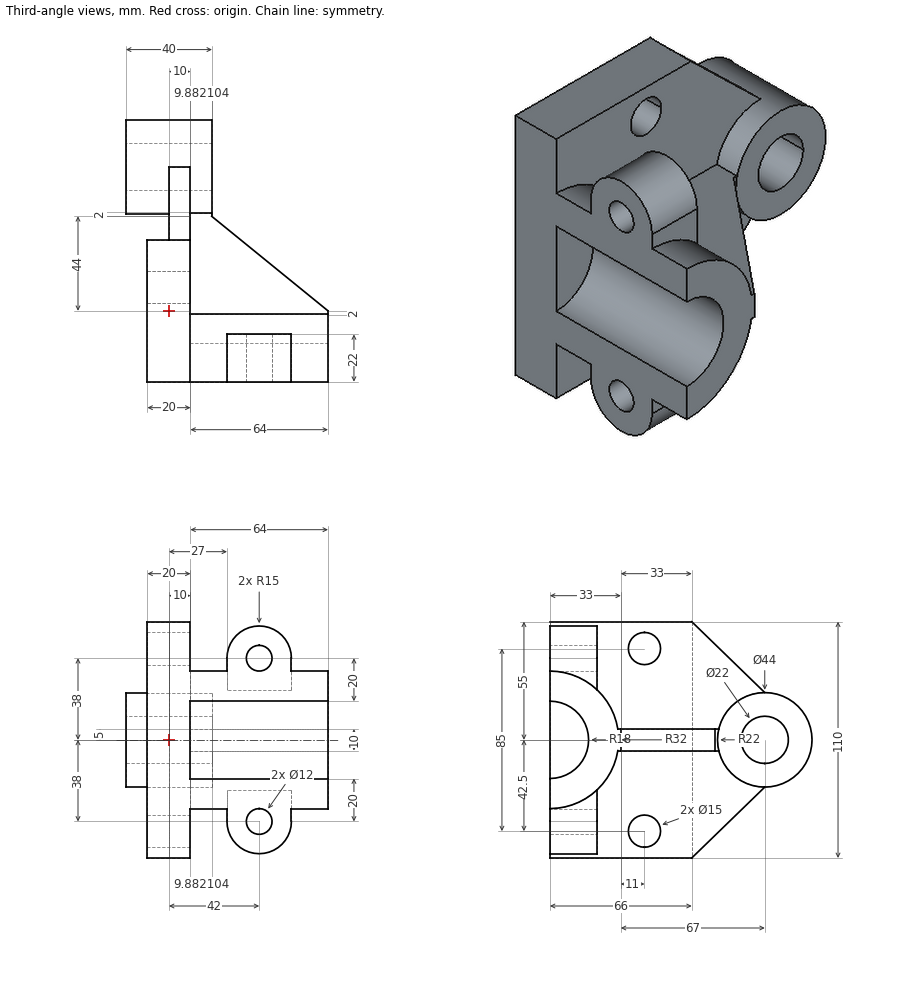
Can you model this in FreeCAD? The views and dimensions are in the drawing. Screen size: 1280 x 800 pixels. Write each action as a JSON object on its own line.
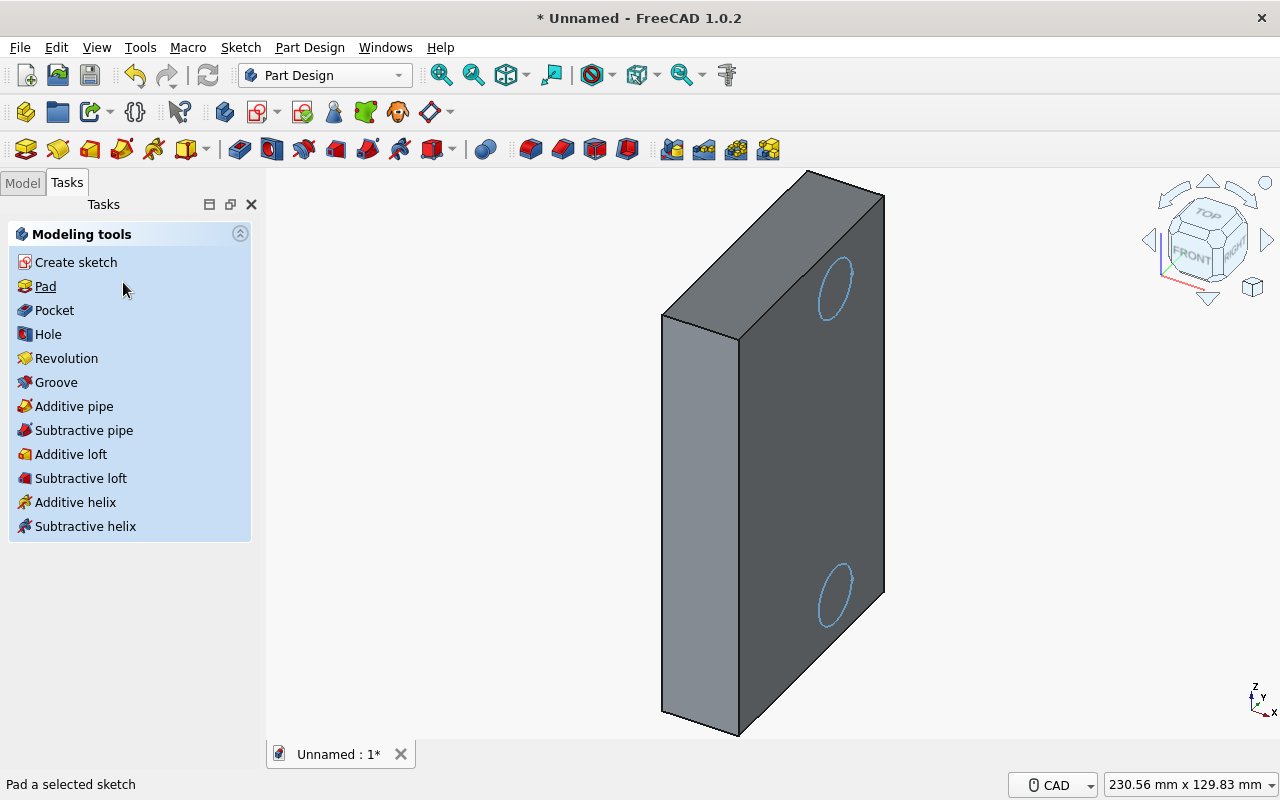
{"action": "left_click", "coordinate": [240, 150]}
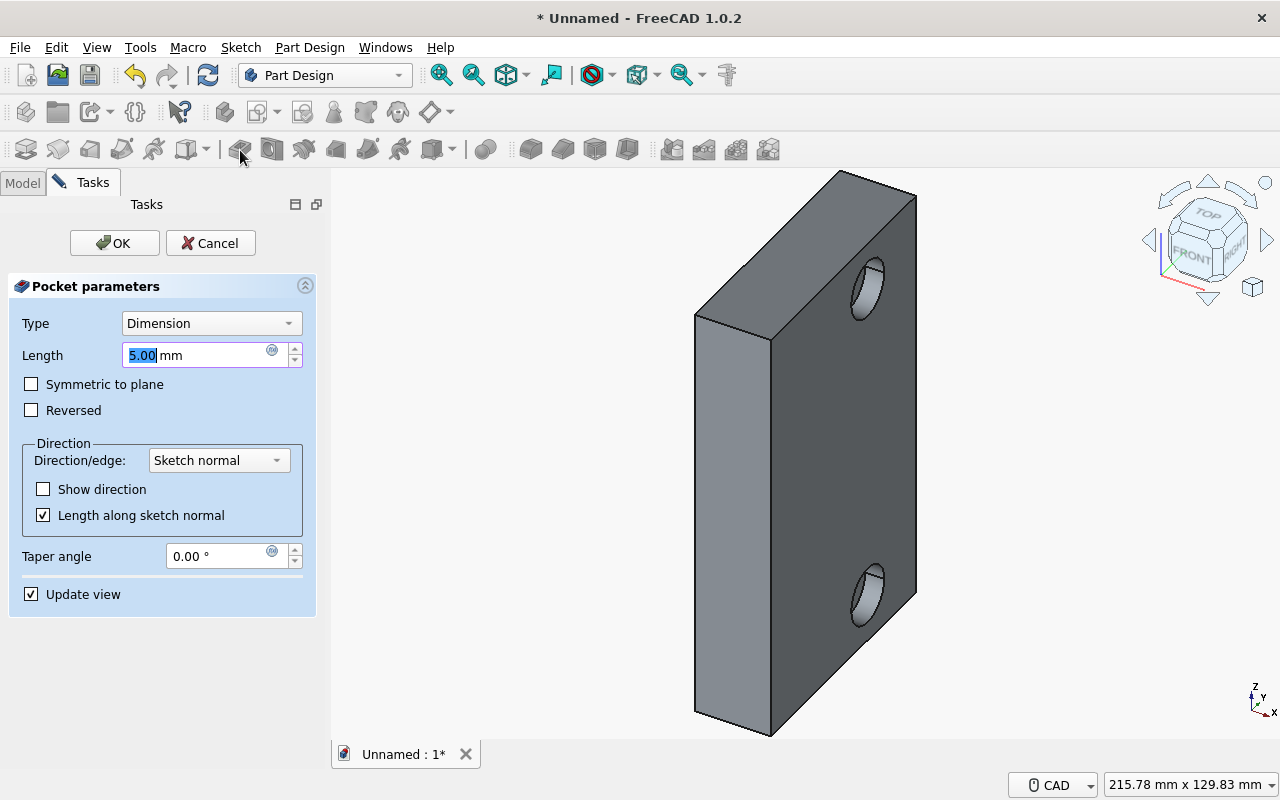
{"action": "type", "text": "20"}
{"action": "key", "text": "Tab"}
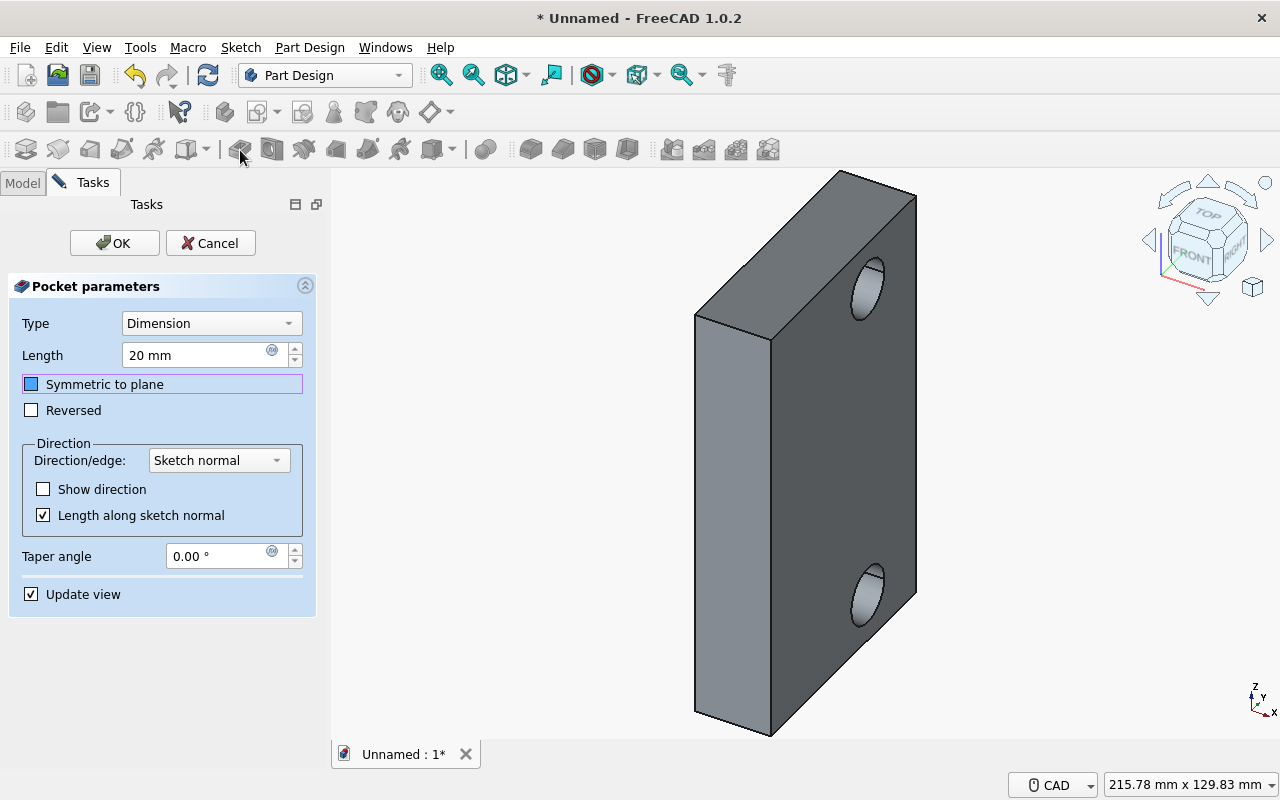
{"action": "left_click", "coordinate": [115, 243]}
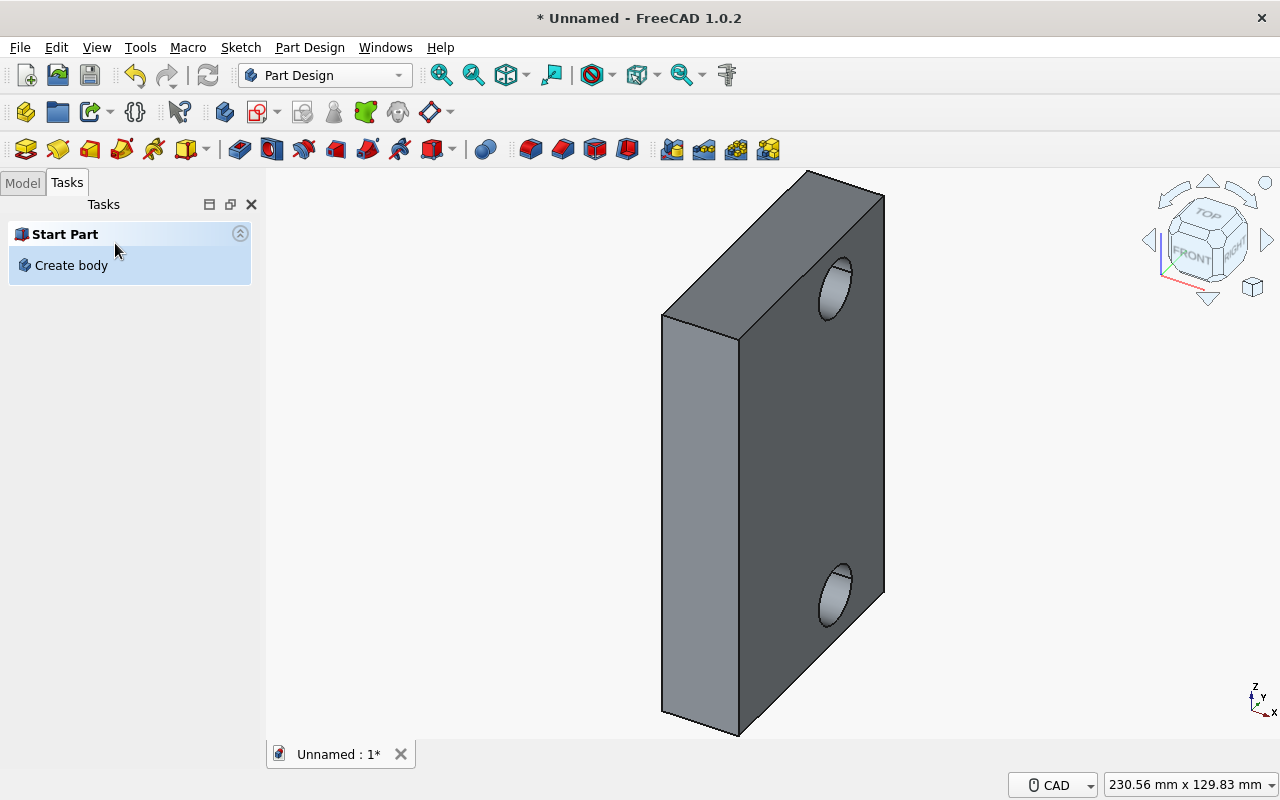
{"action": "left_click", "coordinate": [811, 465]}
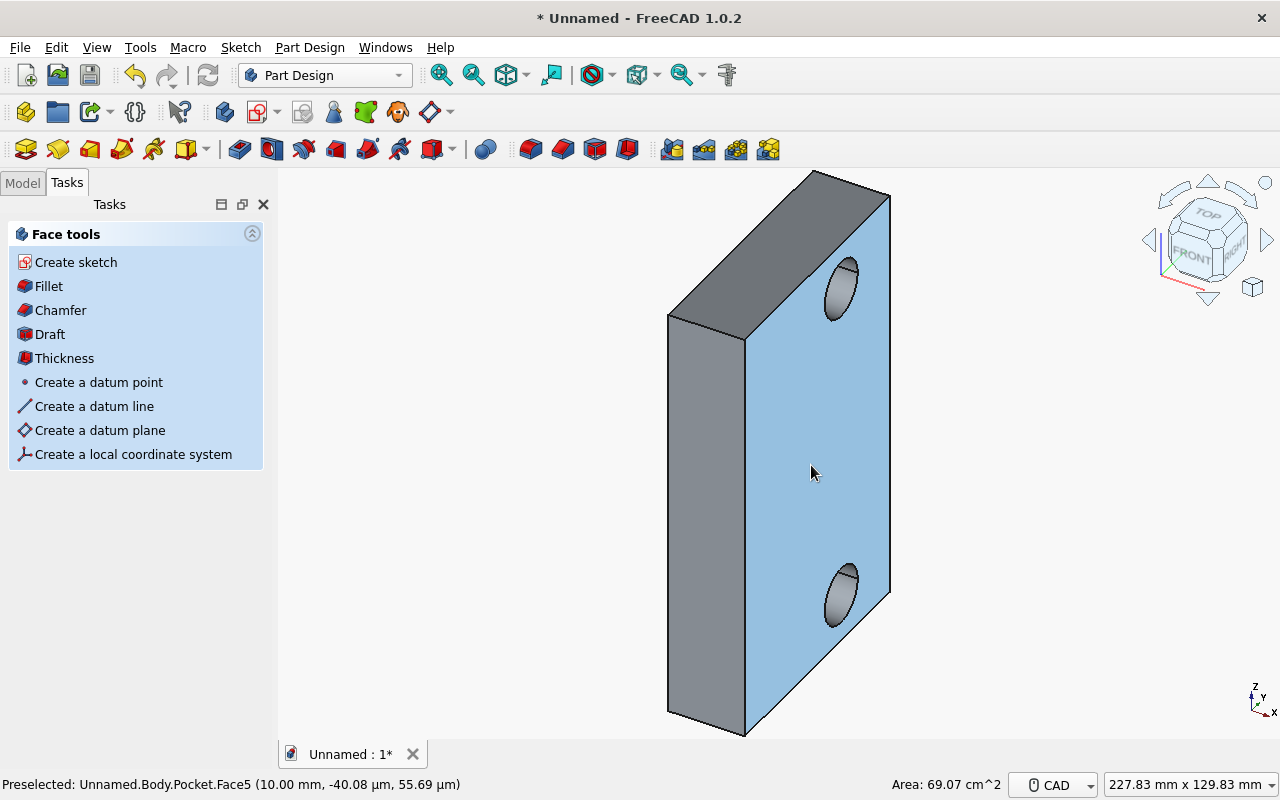
{"action": "left_click", "coordinate": [258, 112]}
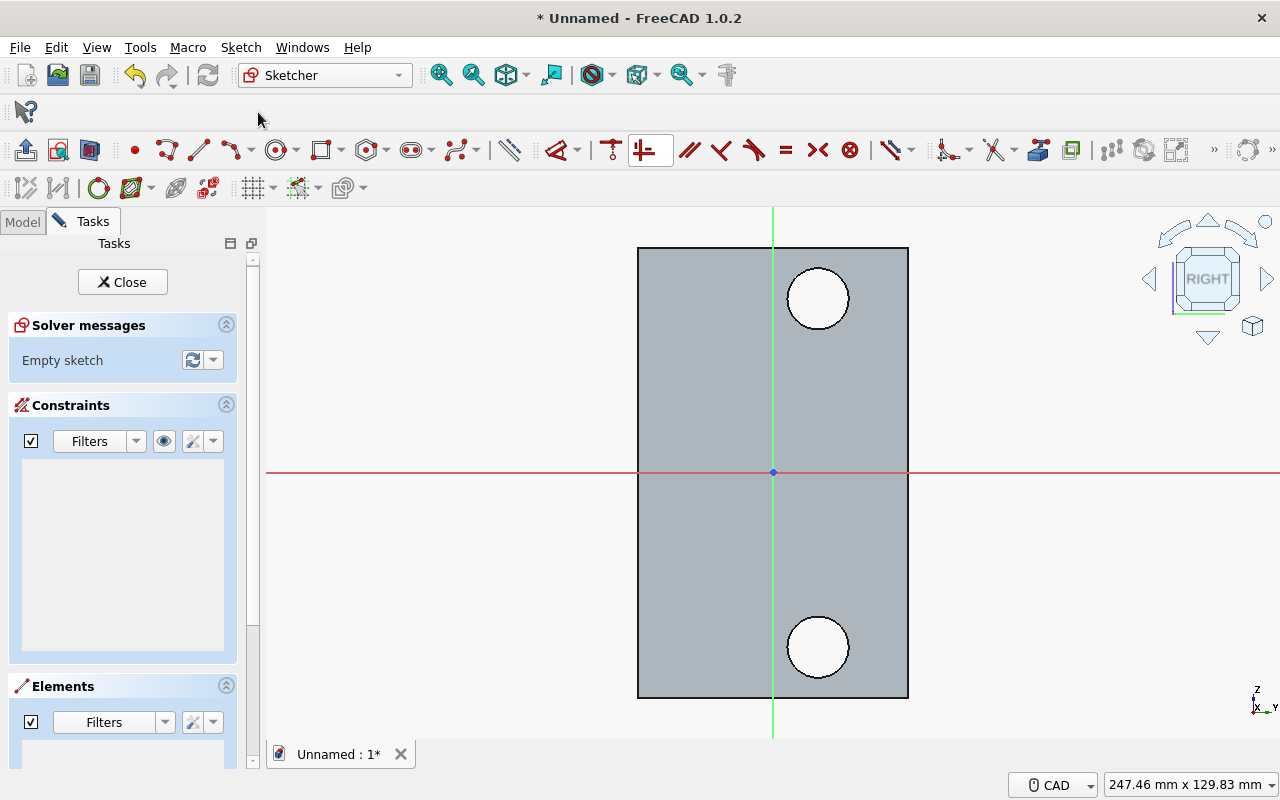
{"action": "key", "text": "g l"}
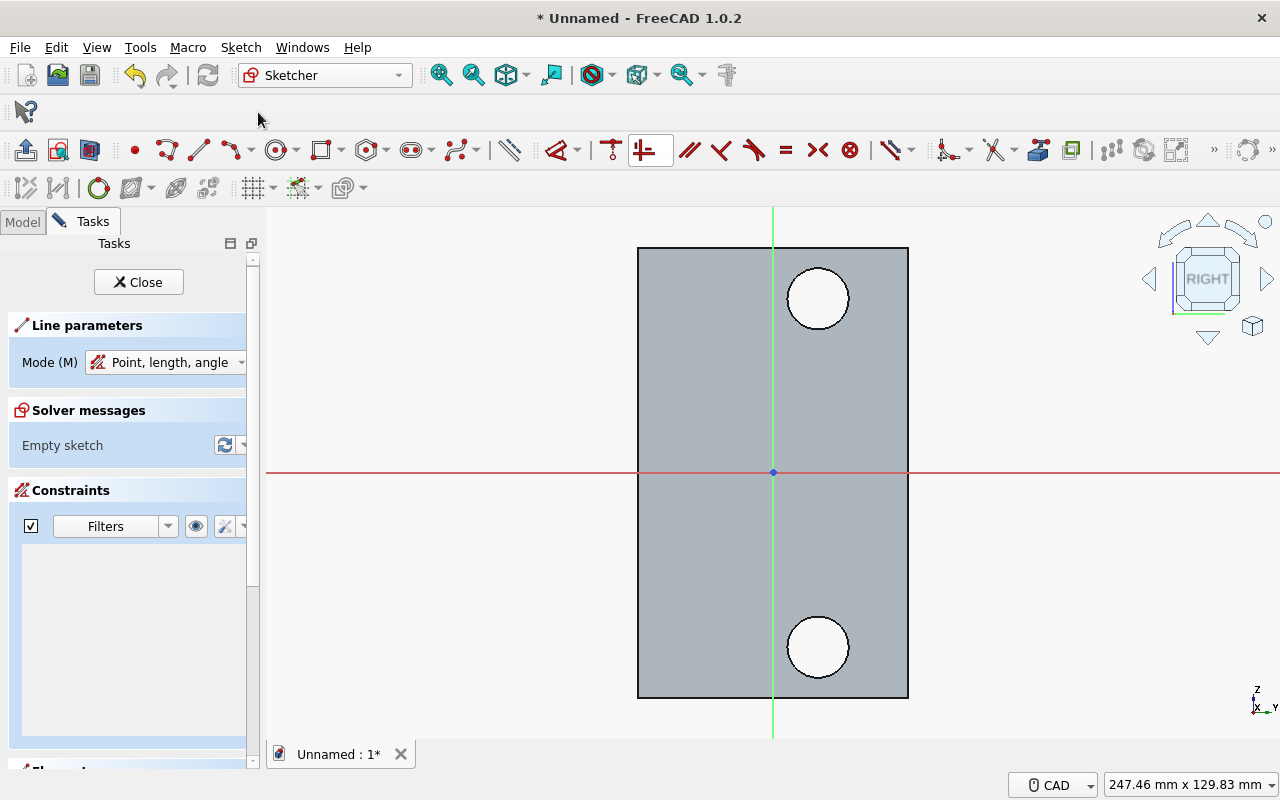
{"action": "left_click", "coordinate": [638, 342]}
{"action": "left_click", "coordinate": [638, 399]}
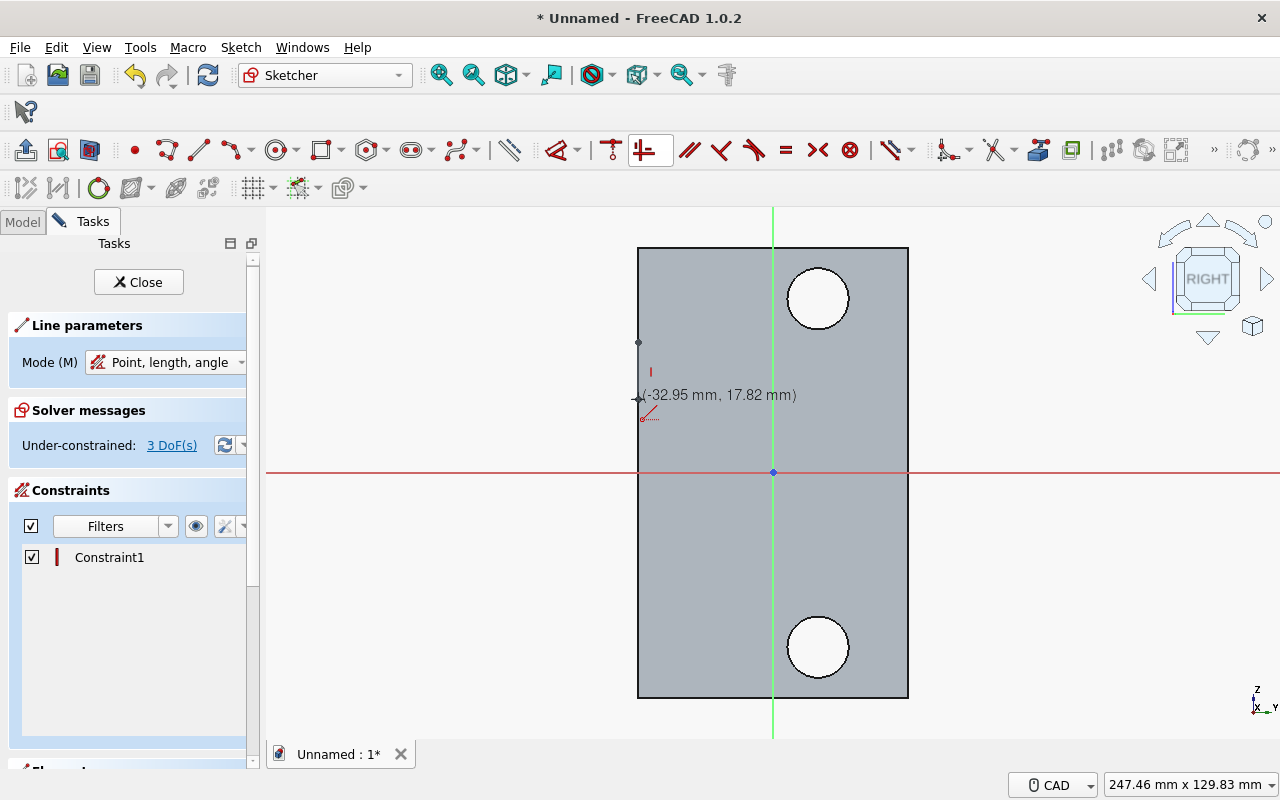
{"action": "left_click", "coordinate": [638, 547]}
{"action": "left_click", "coordinate": [638, 604]}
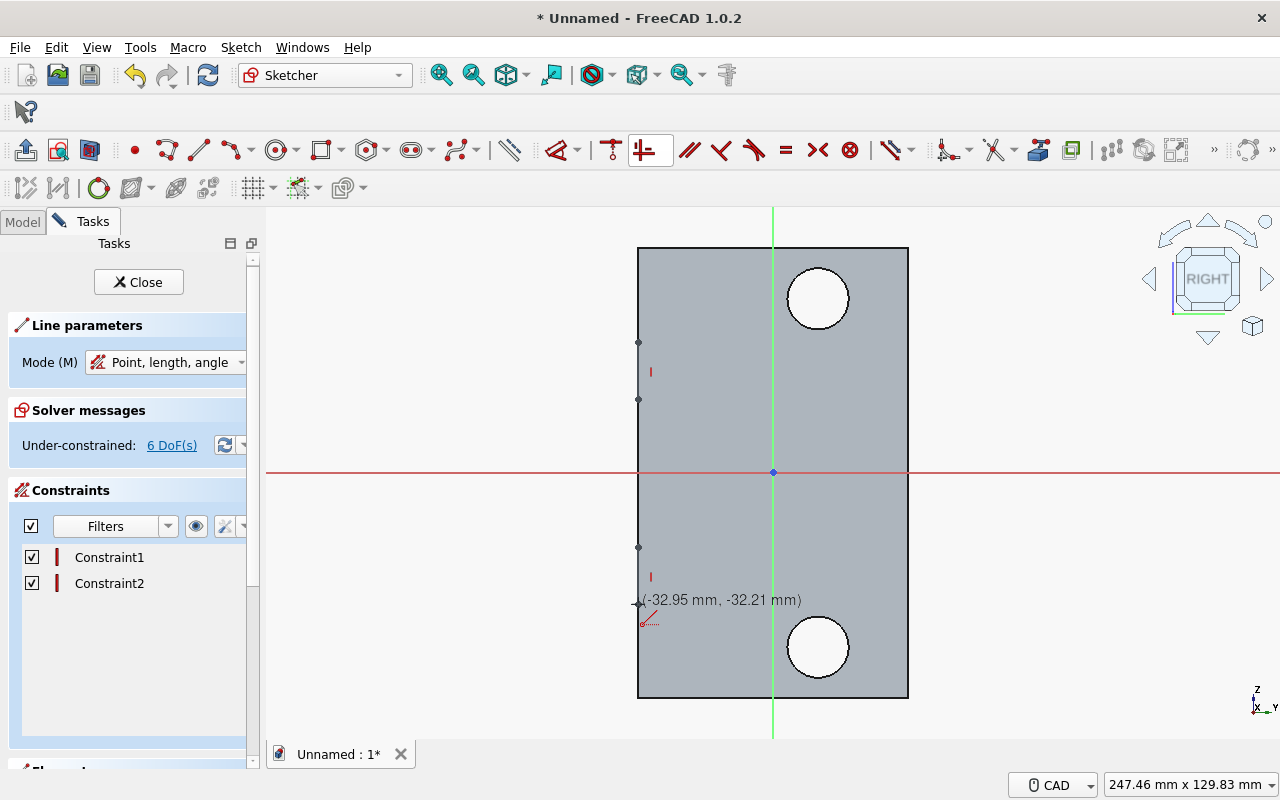
{"action": "key", "text": "g 3 a"}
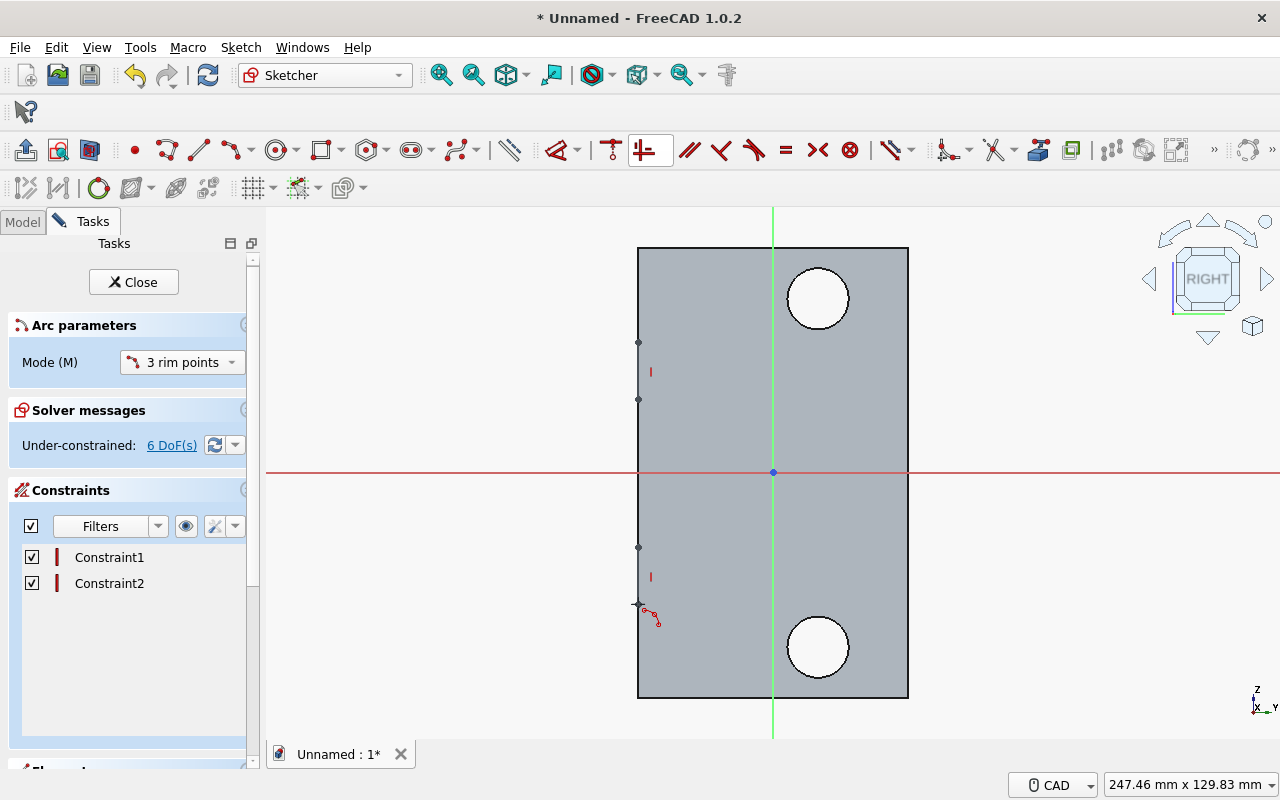
{"action": "left_click", "coordinate": [638, 400]}
{"action": "left_click", "coordinate": [638, 548]}
{"action": "left_click", "coordinate": [708, 496]}